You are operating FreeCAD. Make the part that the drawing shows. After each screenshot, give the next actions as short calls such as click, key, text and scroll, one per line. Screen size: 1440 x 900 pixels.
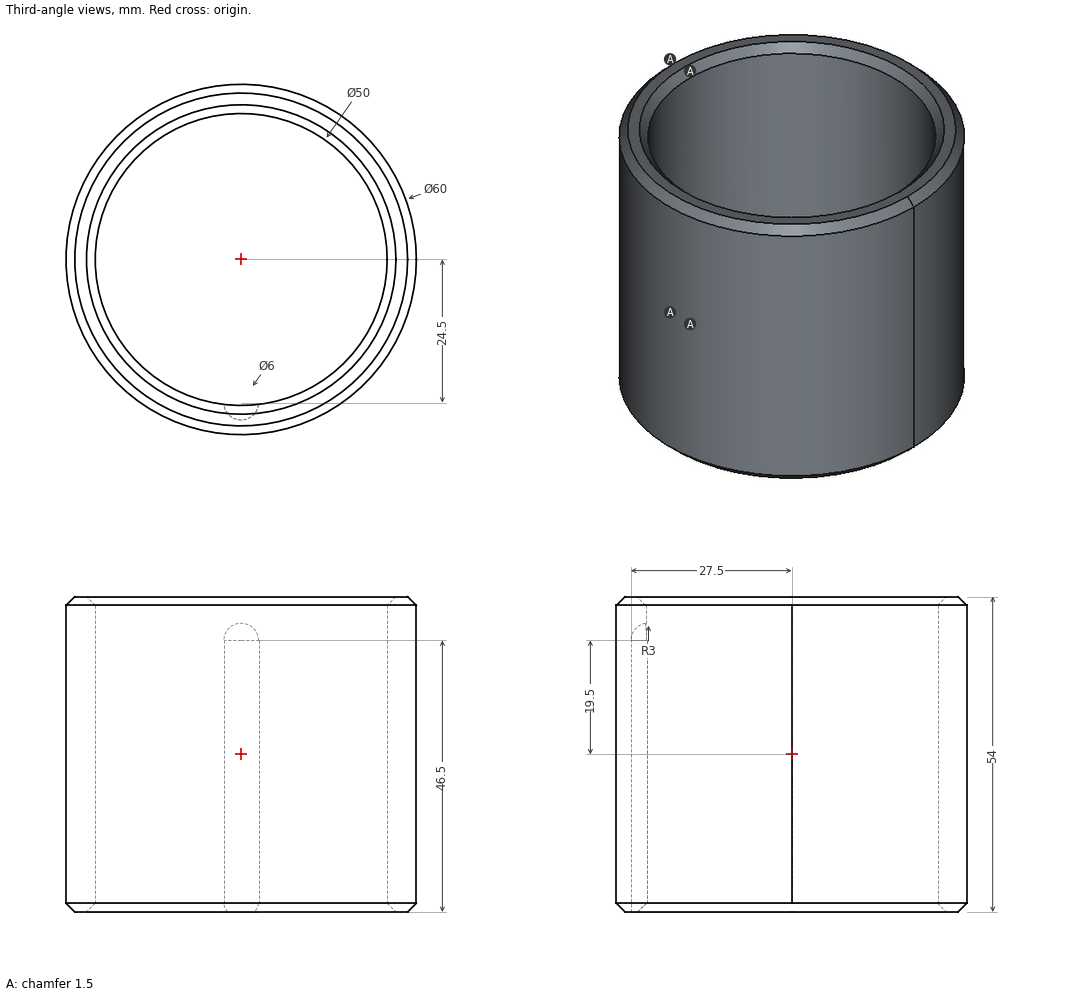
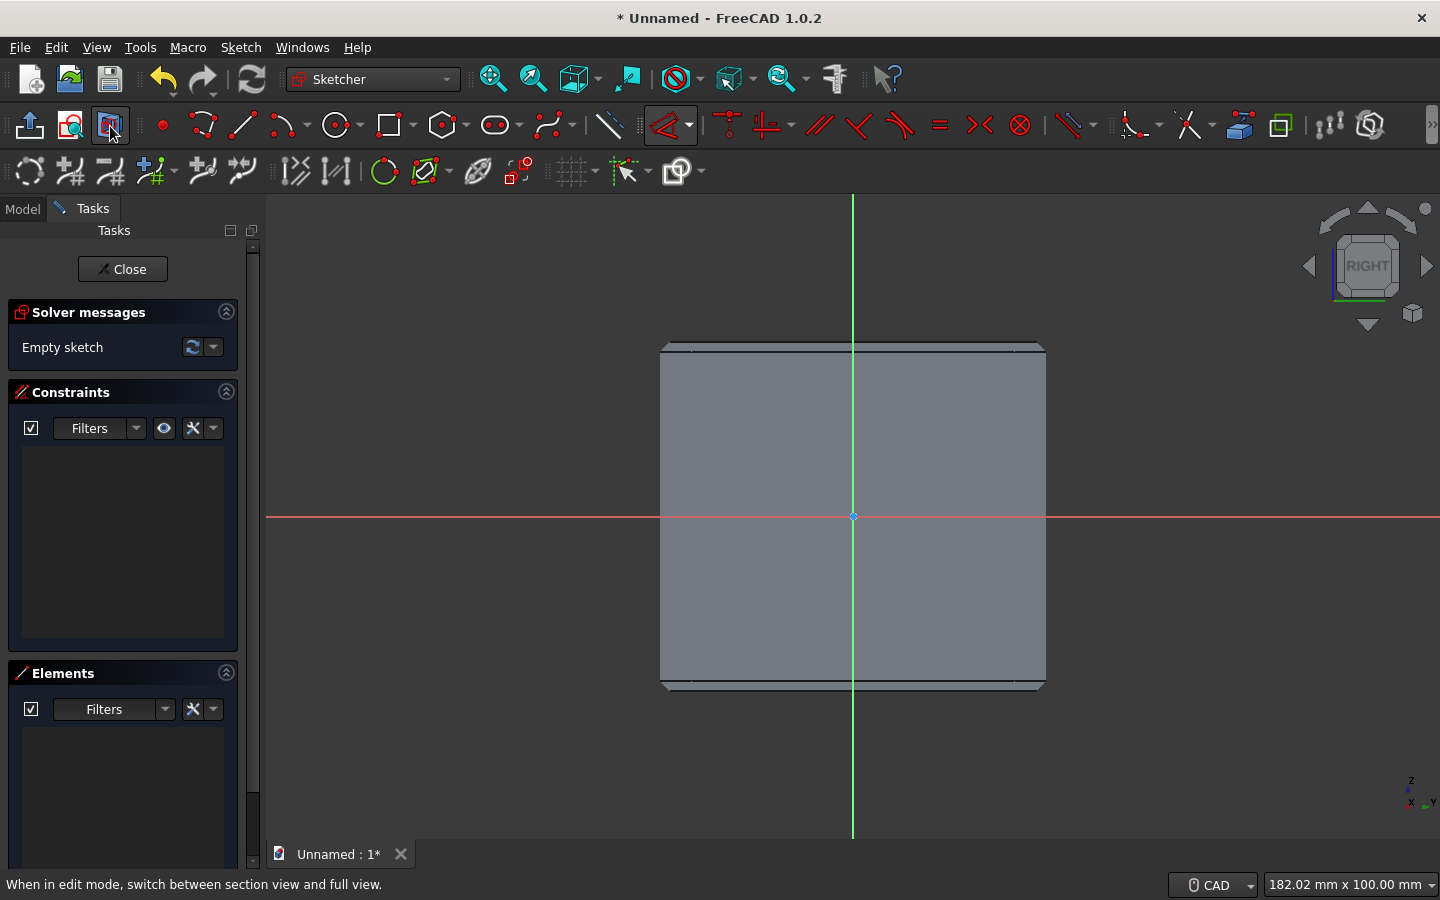
scroll(679, 370, up, 13)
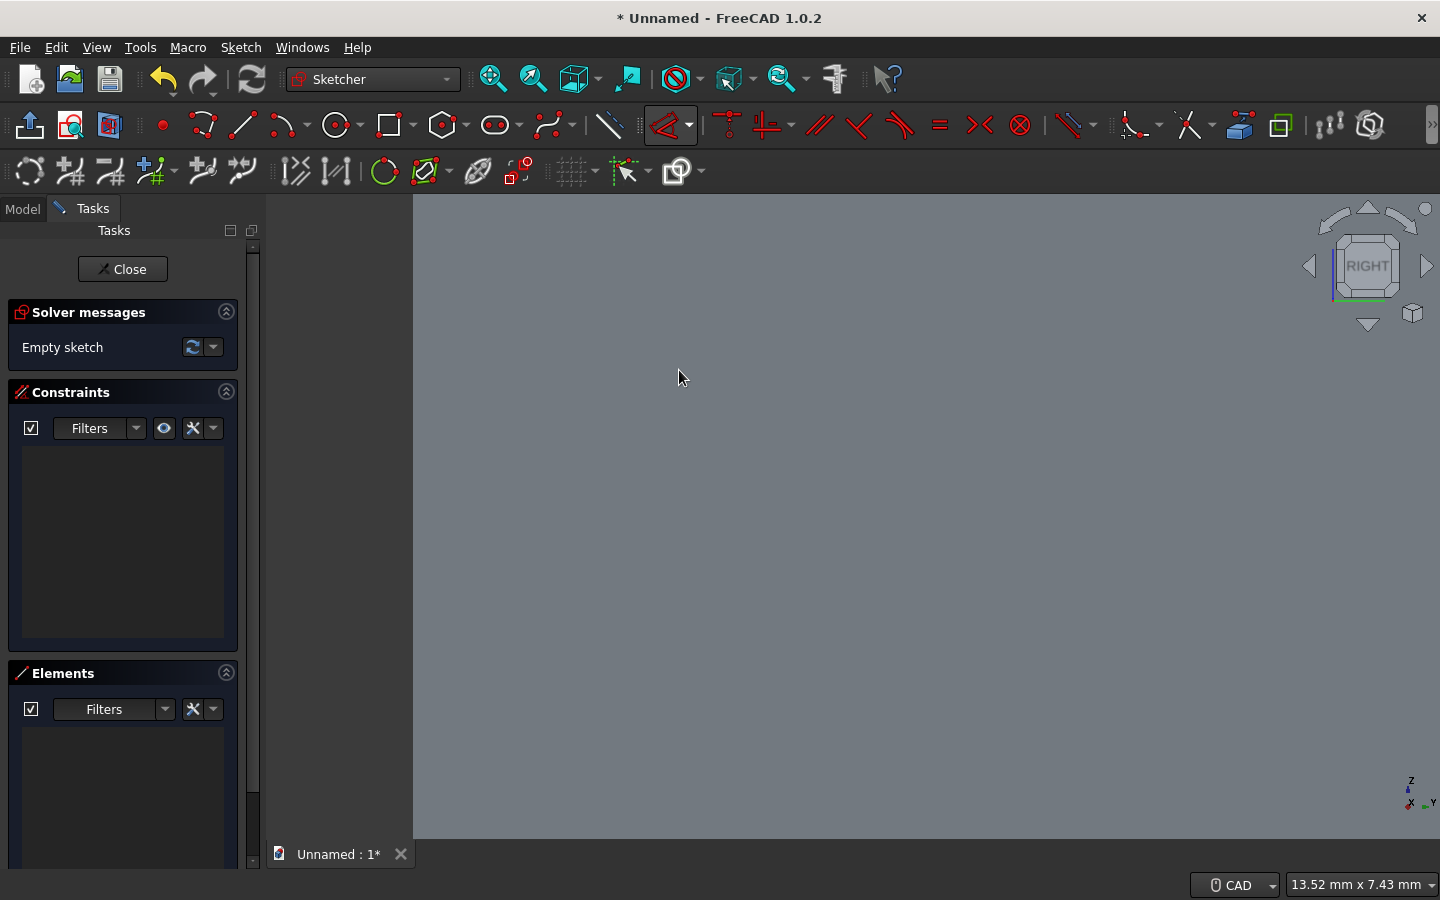
click(244, 126)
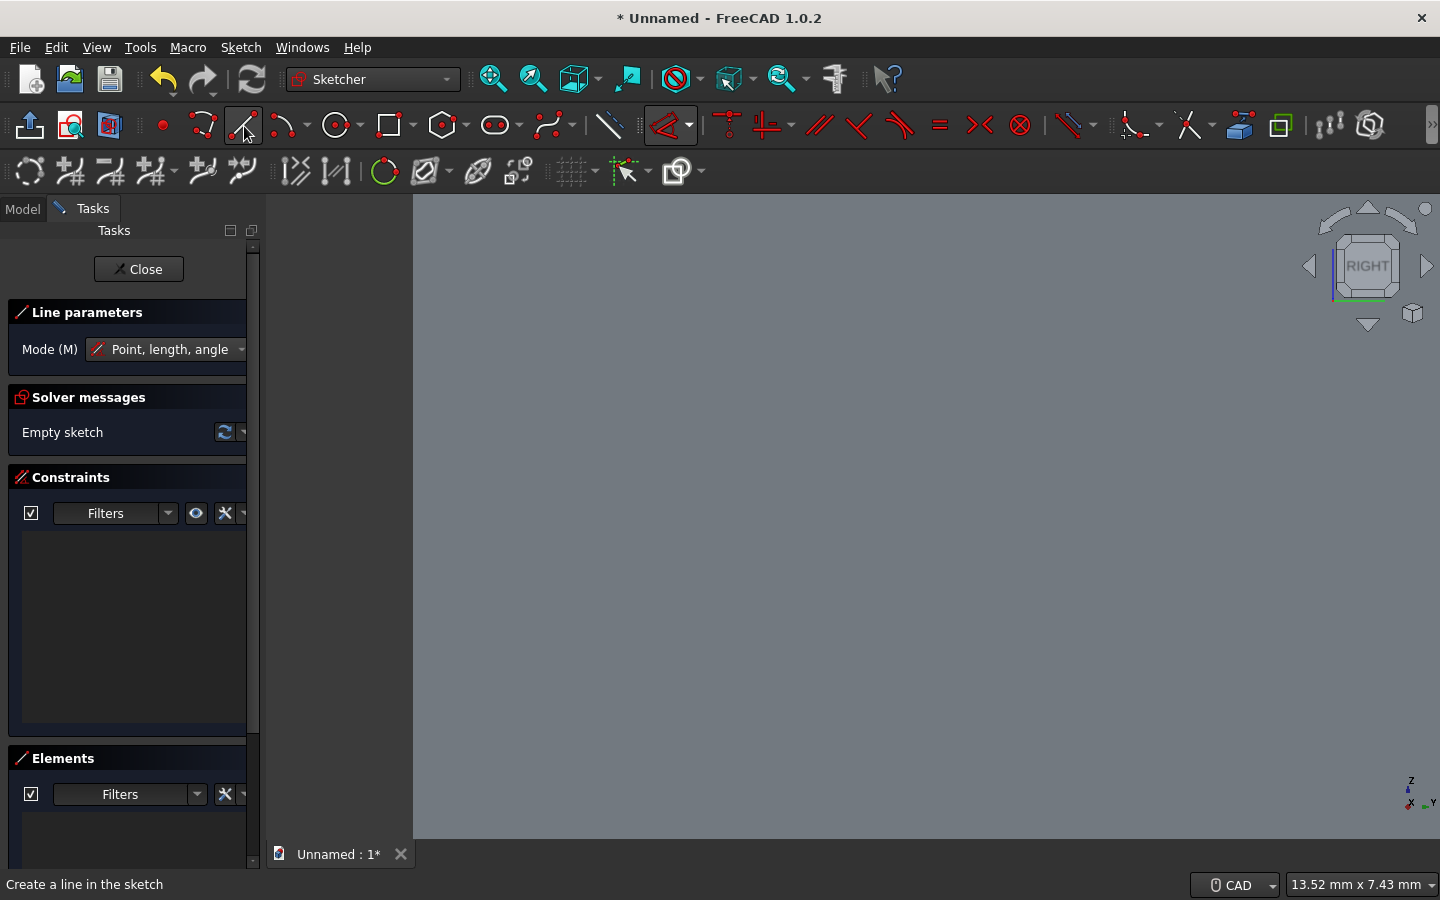
click(629, 646)
click(1150, 646)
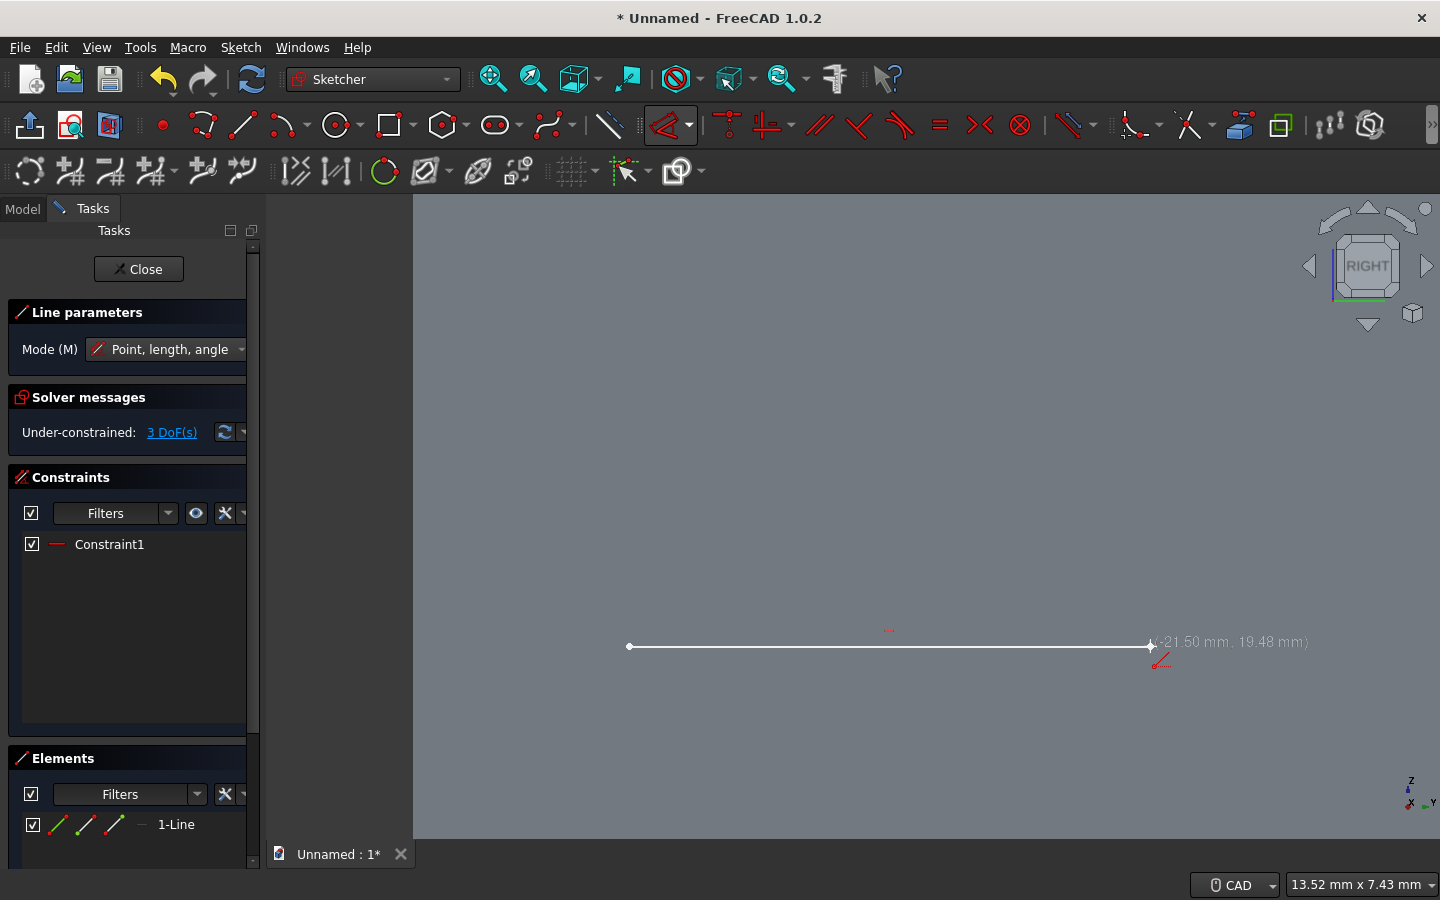
click(310, 126)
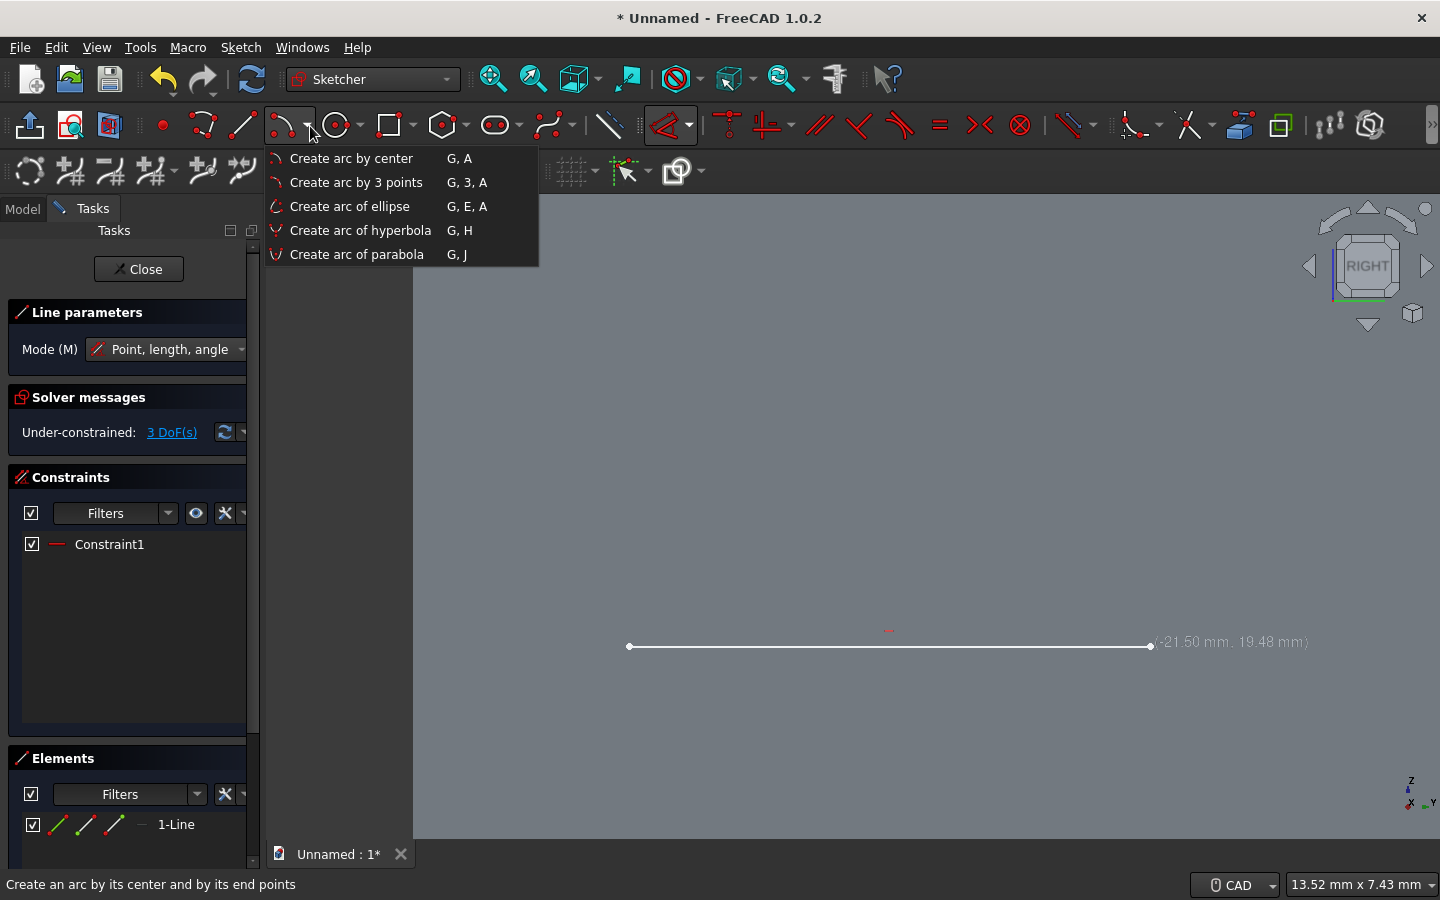
click(402, 182)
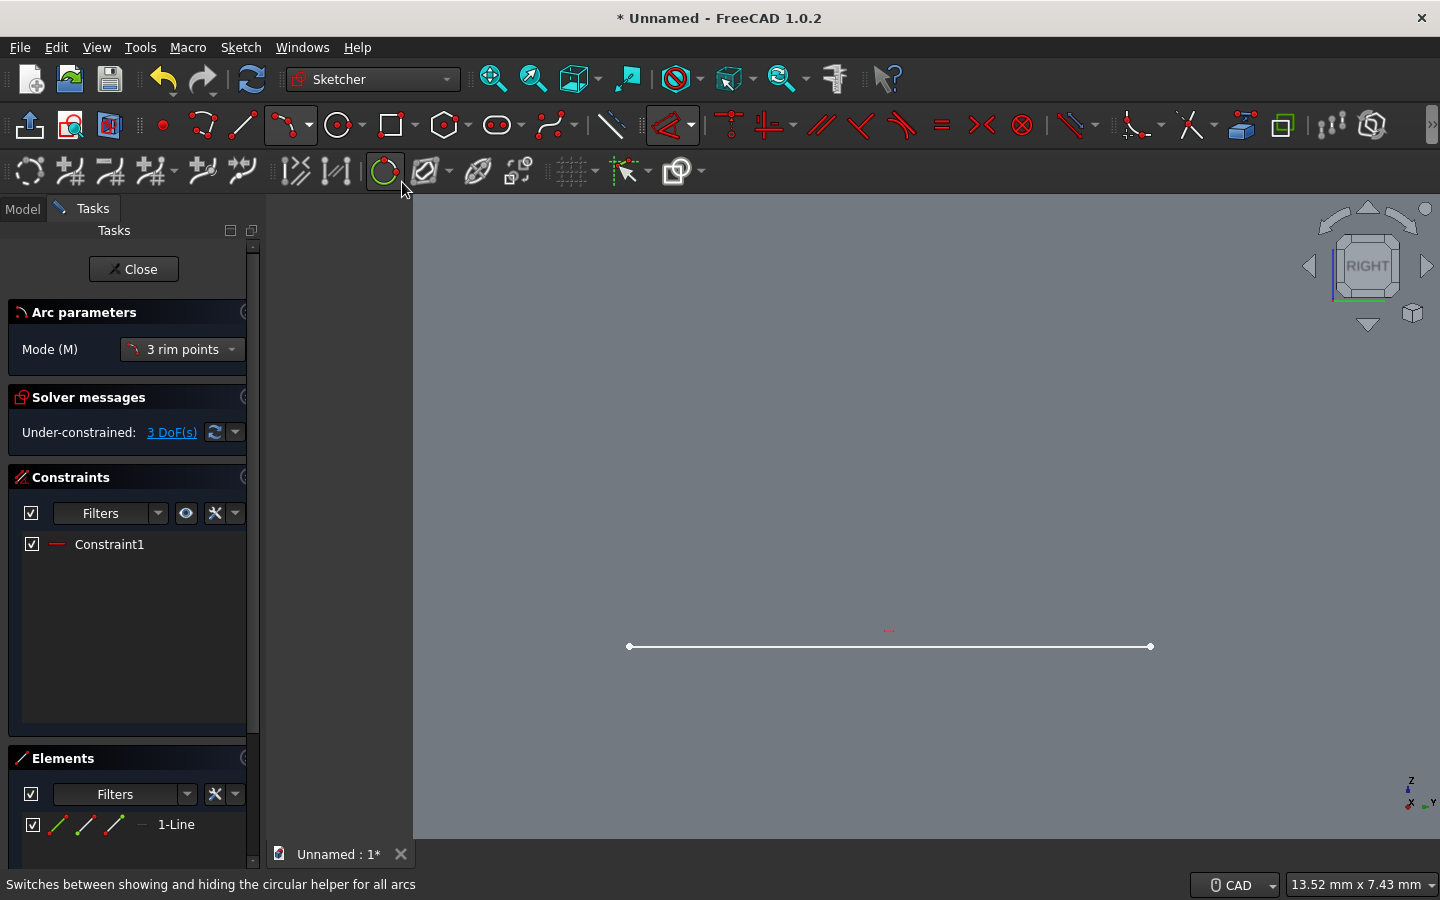
click(1150, 647)
click(629, 647)
click(890, 385)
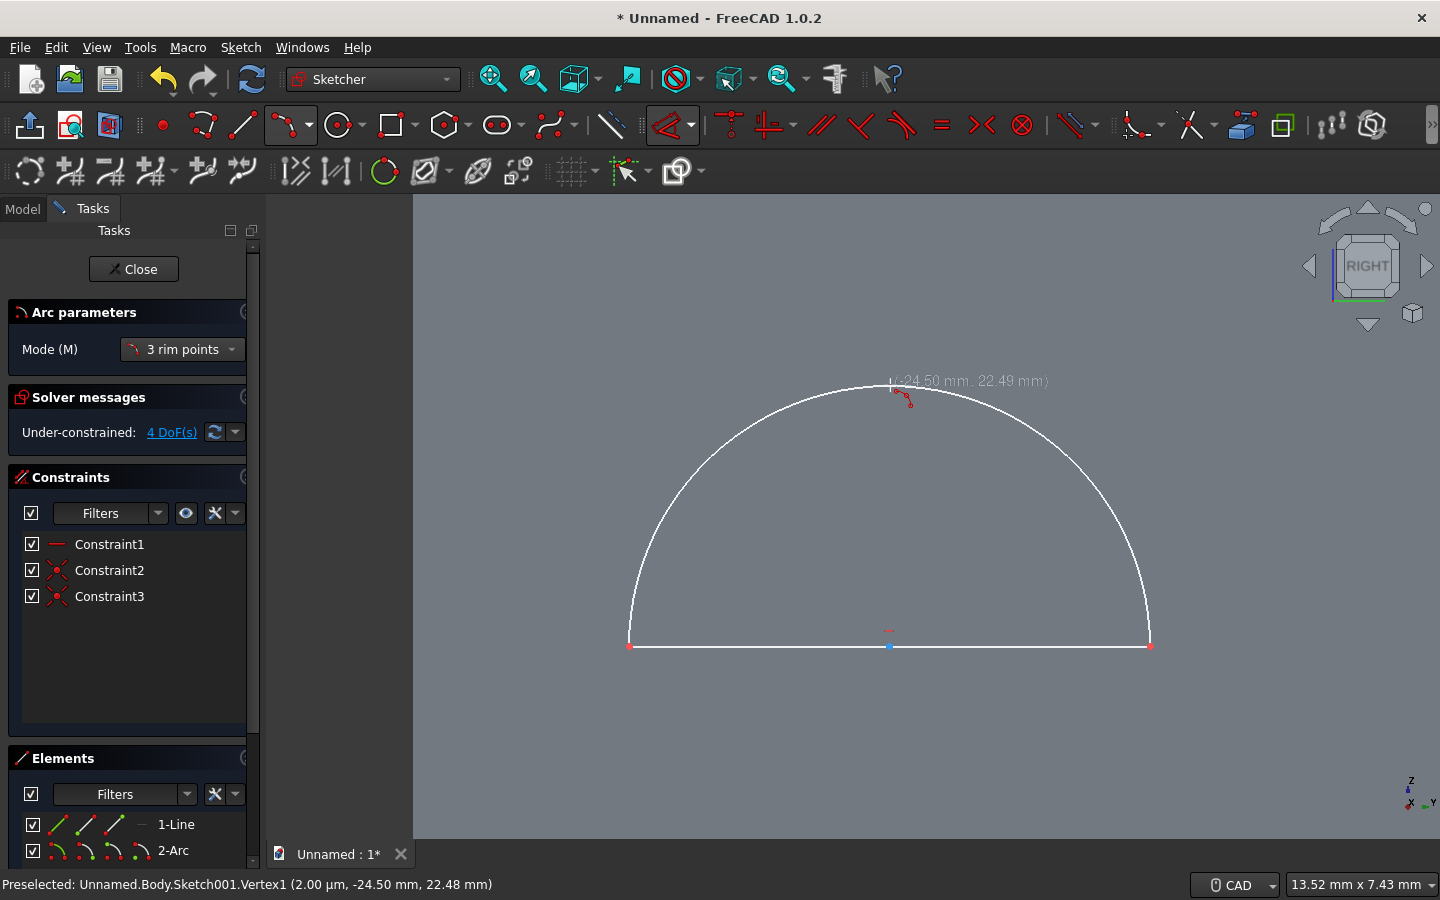
click(244, 126)